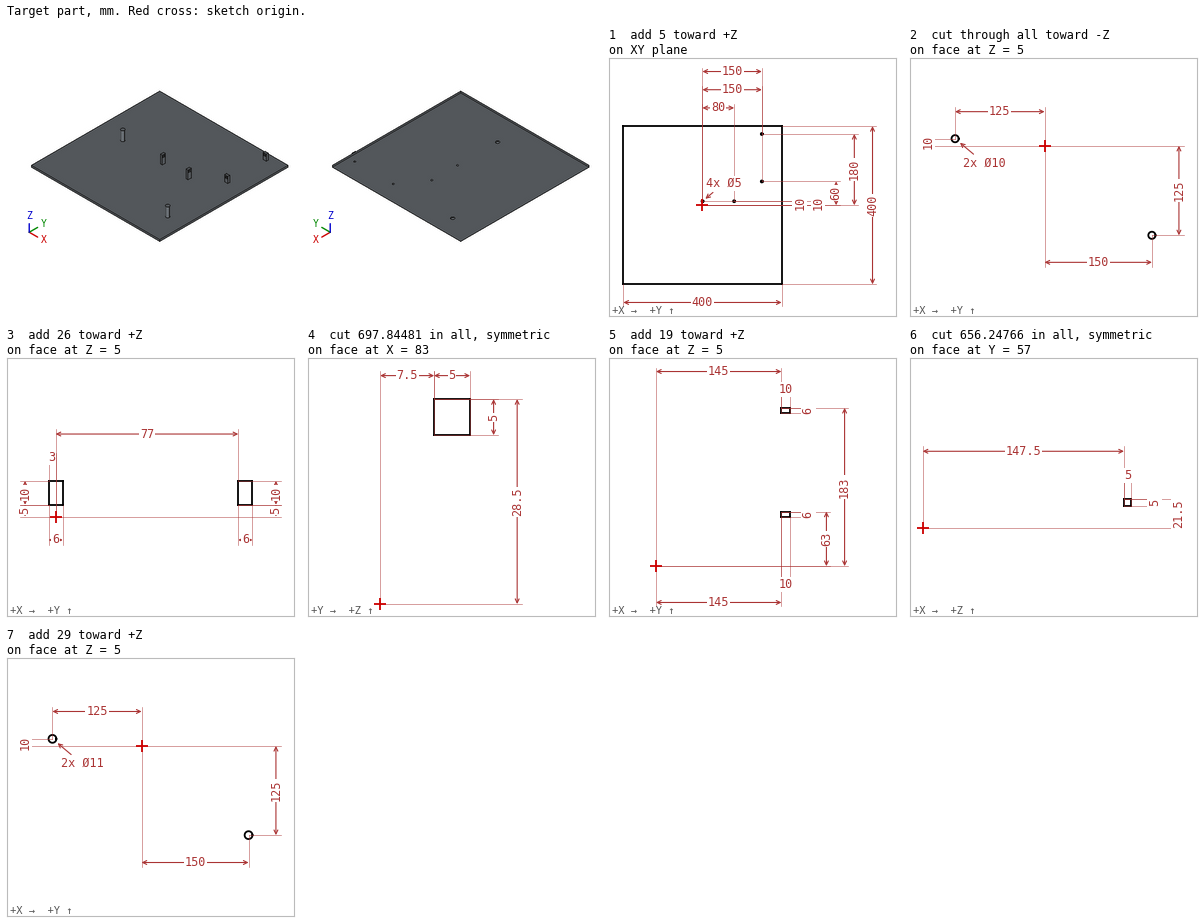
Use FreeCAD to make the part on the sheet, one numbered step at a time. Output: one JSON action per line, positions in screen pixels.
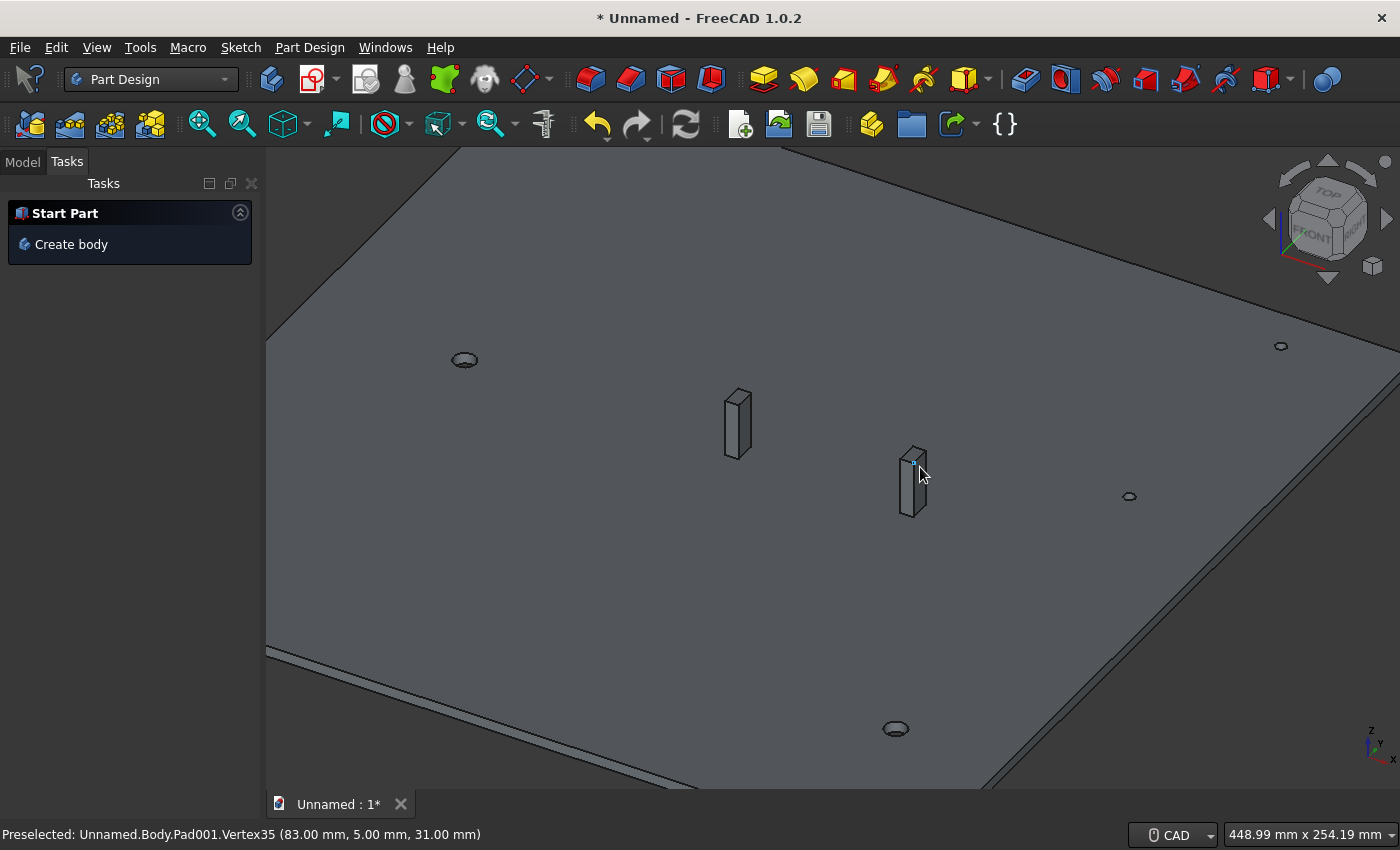
{"action": "left_click", "coordinate": [922, 474]}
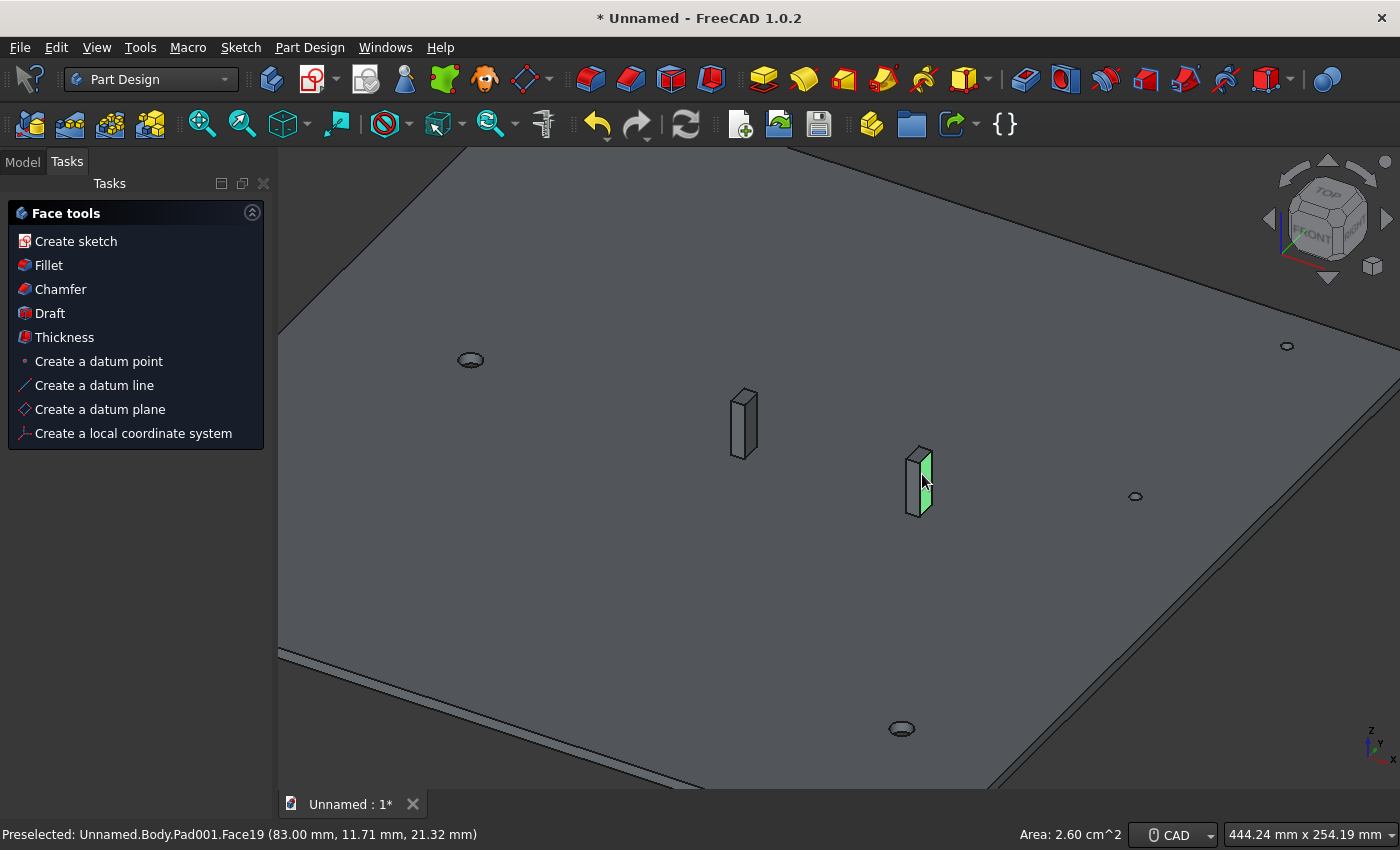
{"action": "left_click", "coordinate": [312, 80]}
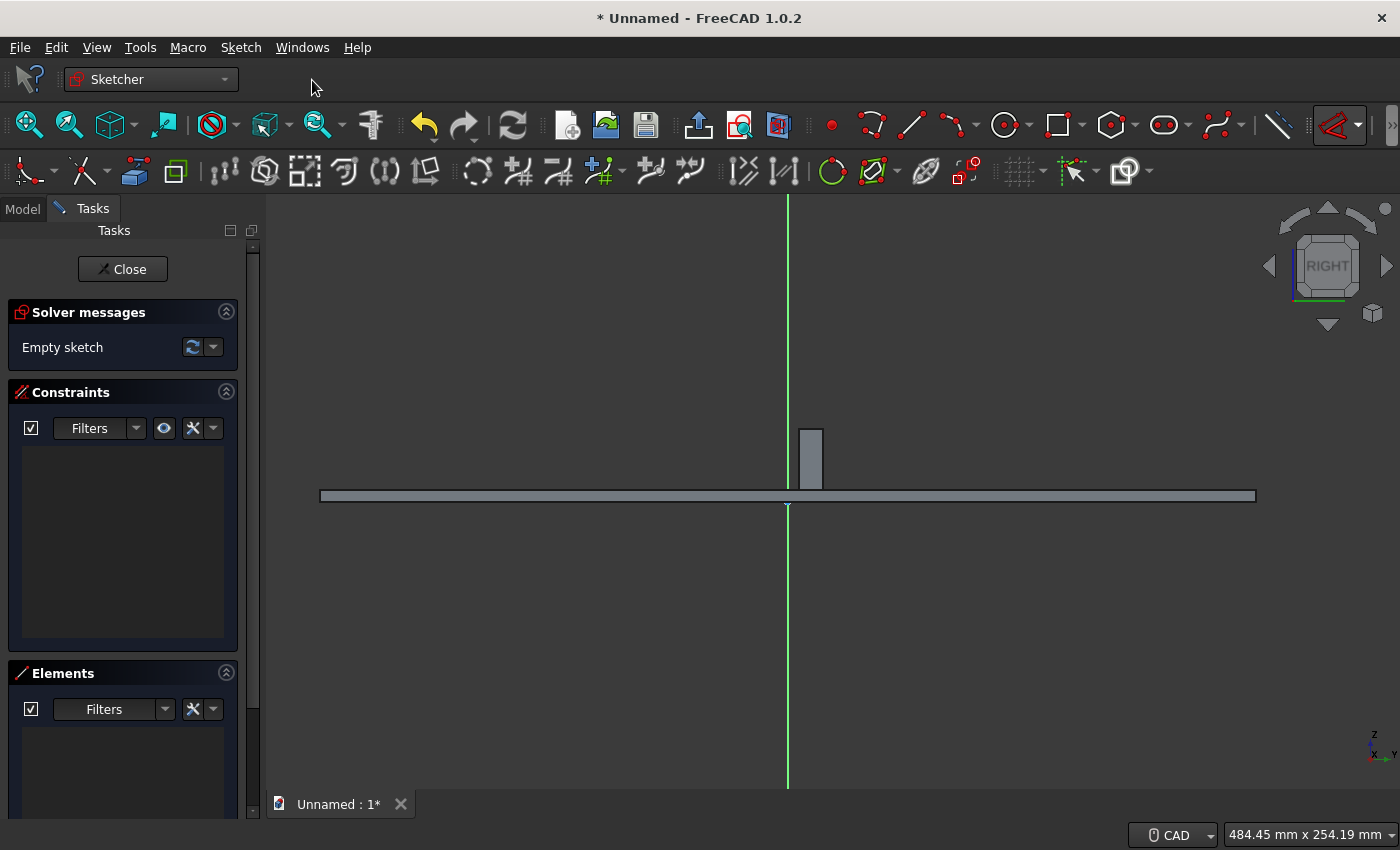
{"action": "scroll", "coordinate": [814, 438], "scroll_direction": "up", "scroll_amount": 15}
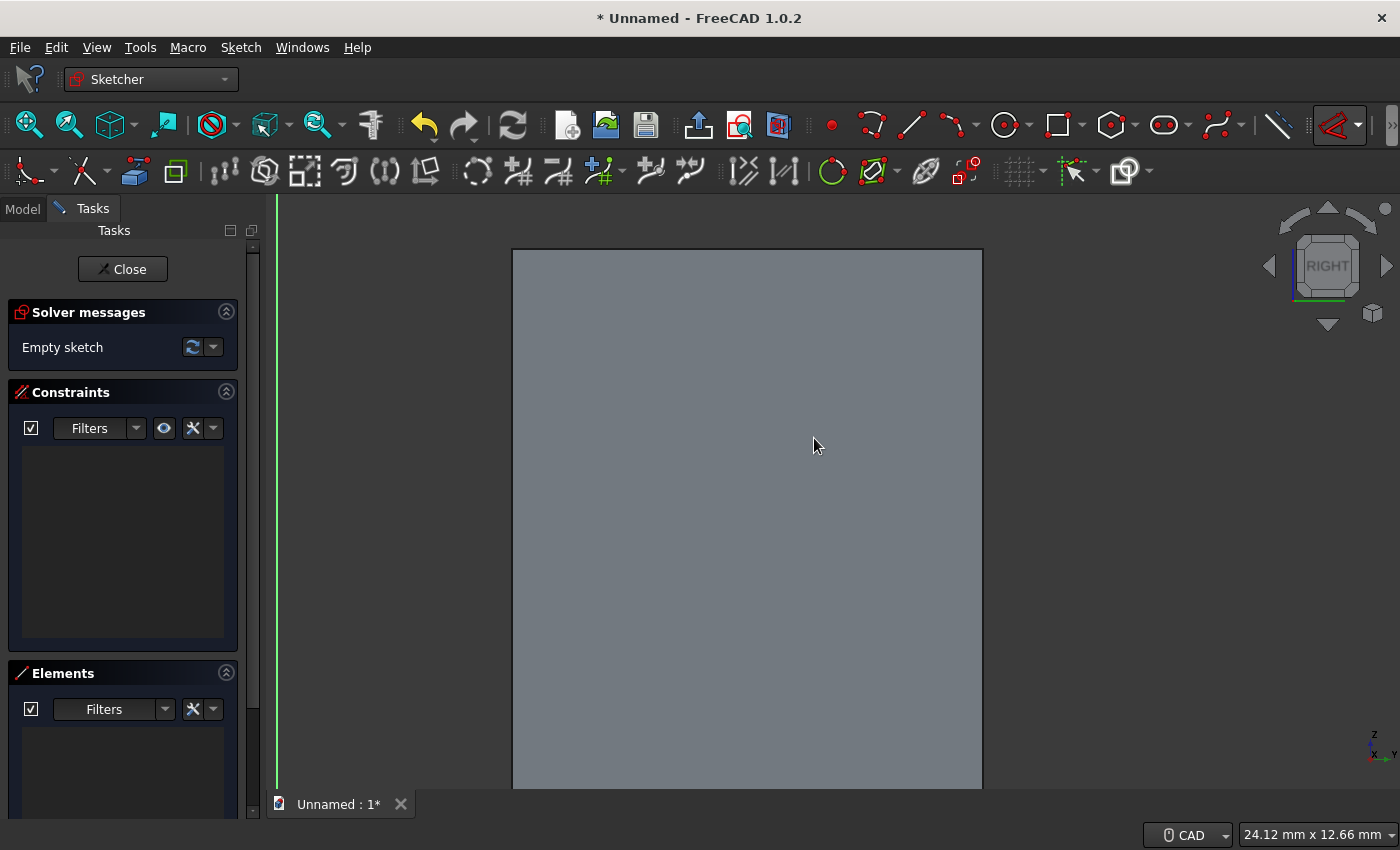
{"action": "scroll", "coordinate": [713, 469], "scroll_direction": "up", "scroll_amount": 2}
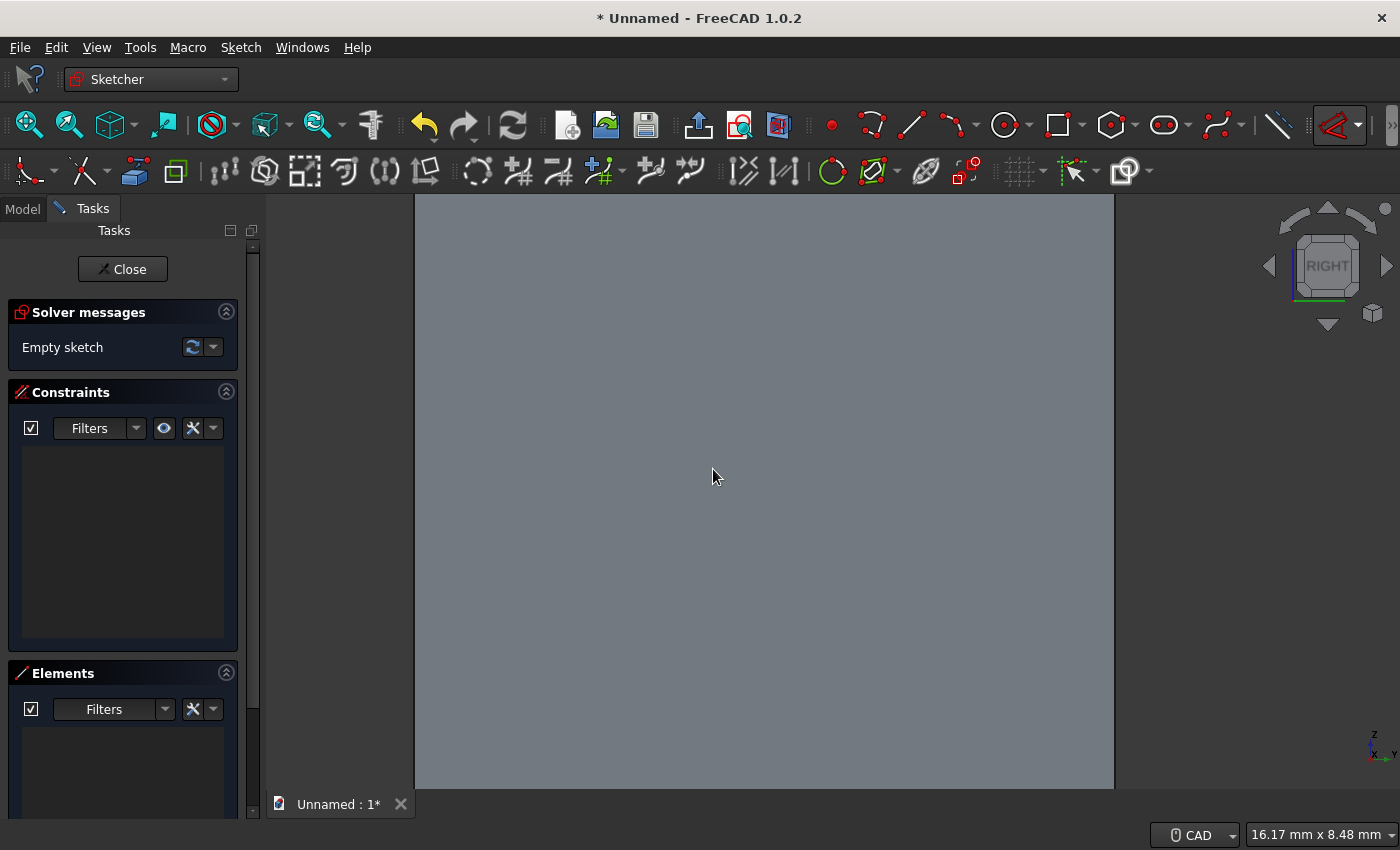
{"action": "key", "text": "g r"}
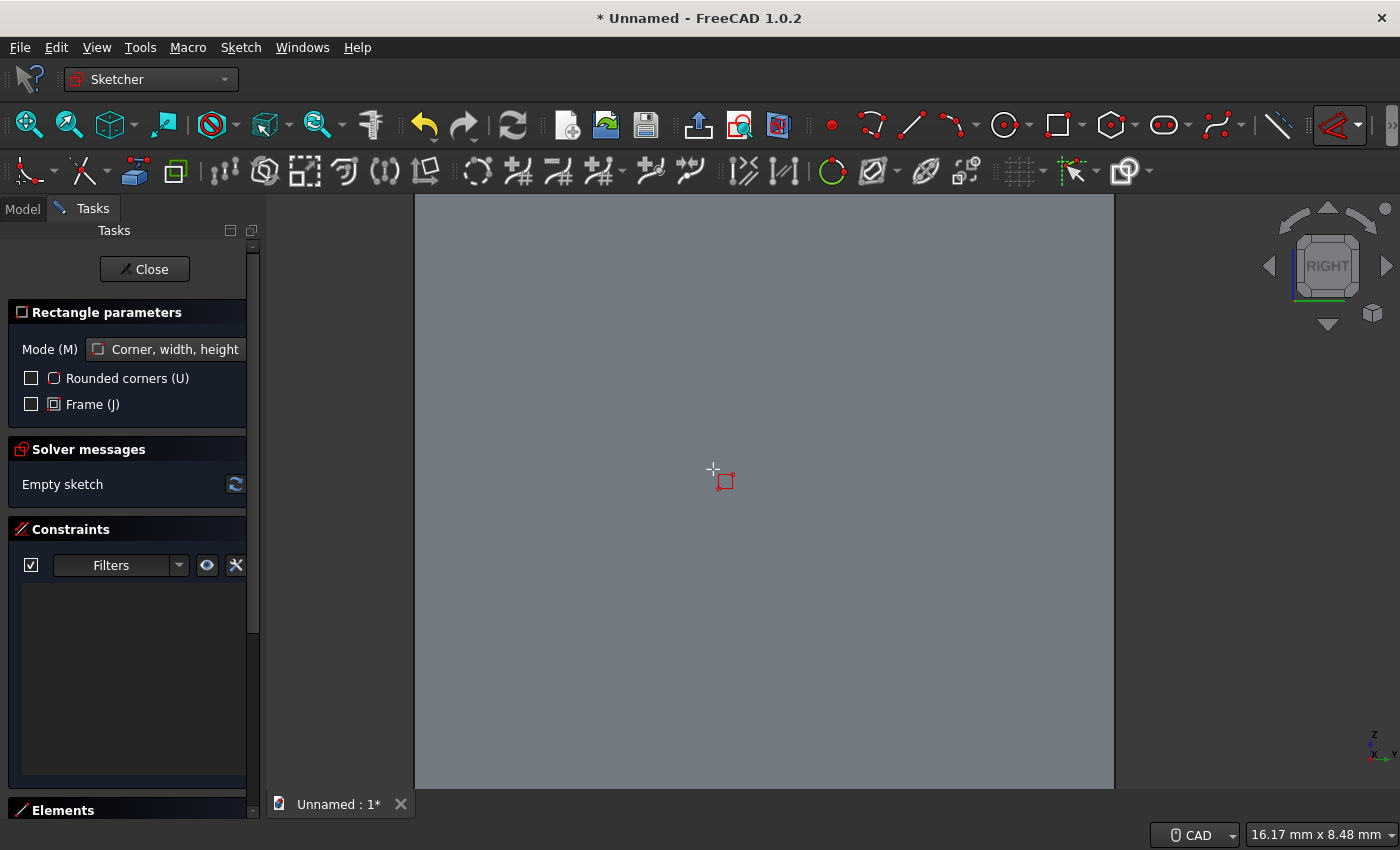
{"action": "left_click", "coordinate": [589, 316]}
{"action": "left_click", "coordinate": [940, 667]}
{"action": "key", "text": "Escape"}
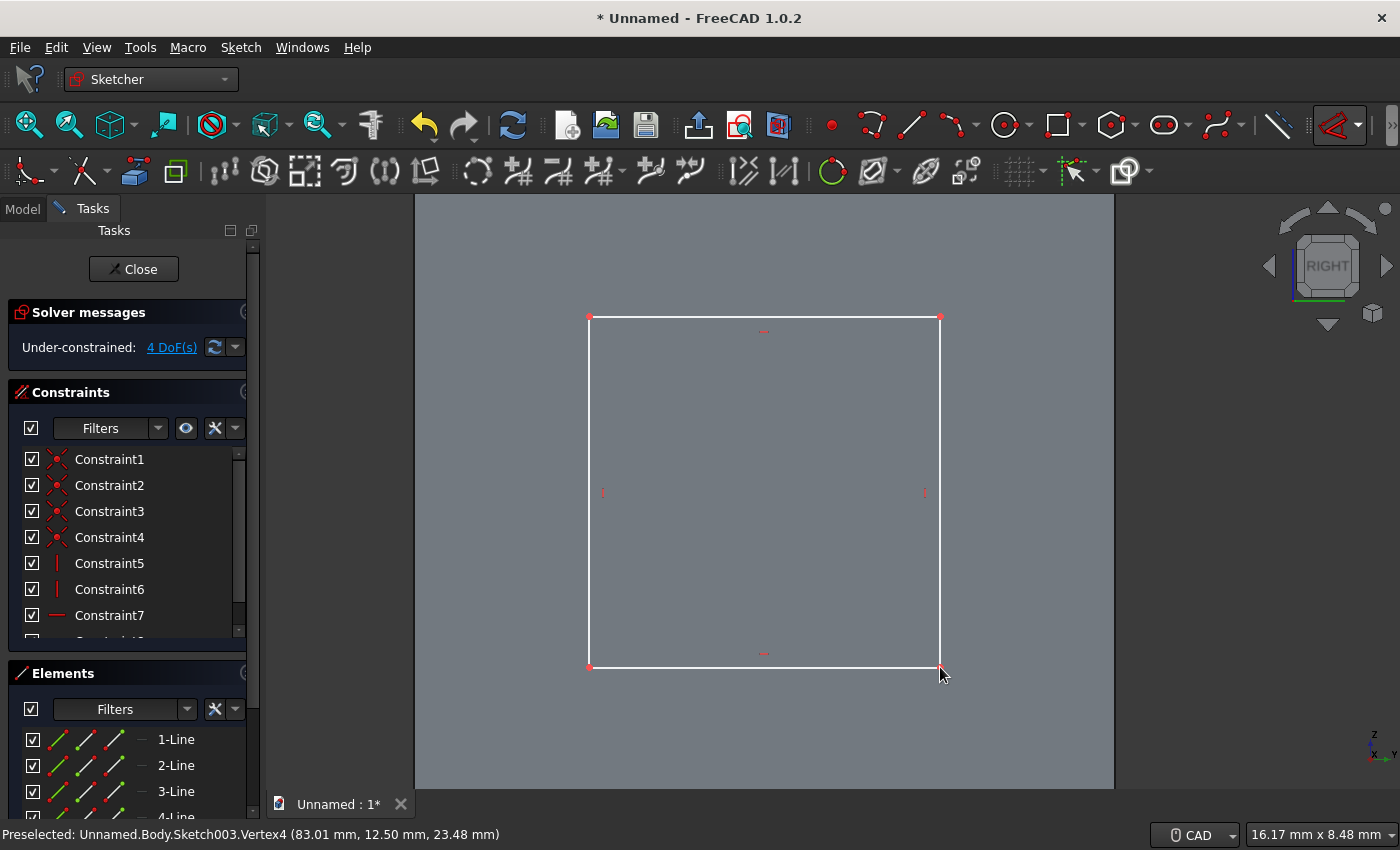
{"action": "left_click", "coordinate": [589, 422]}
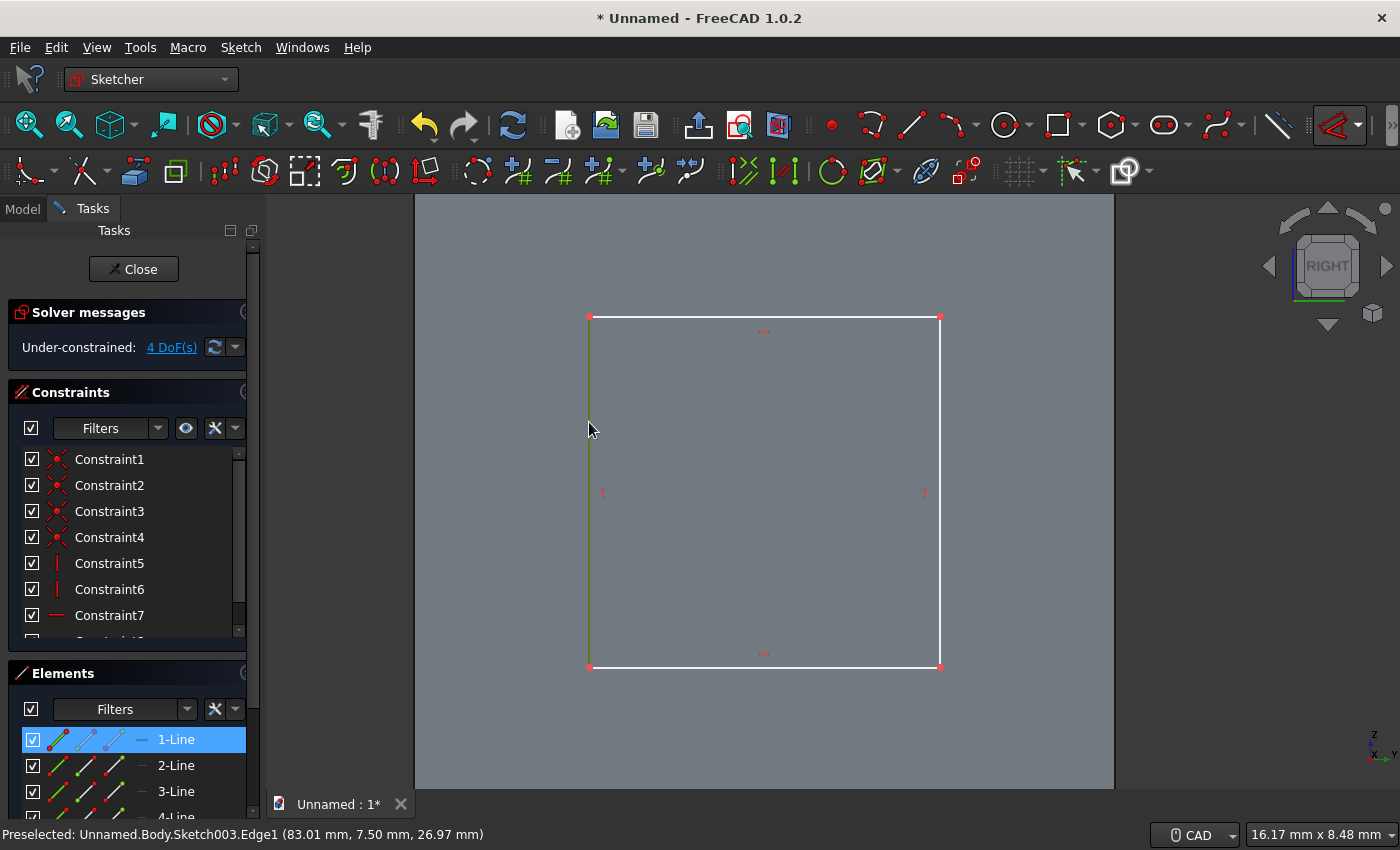
{"action": "key", "text": "i"}